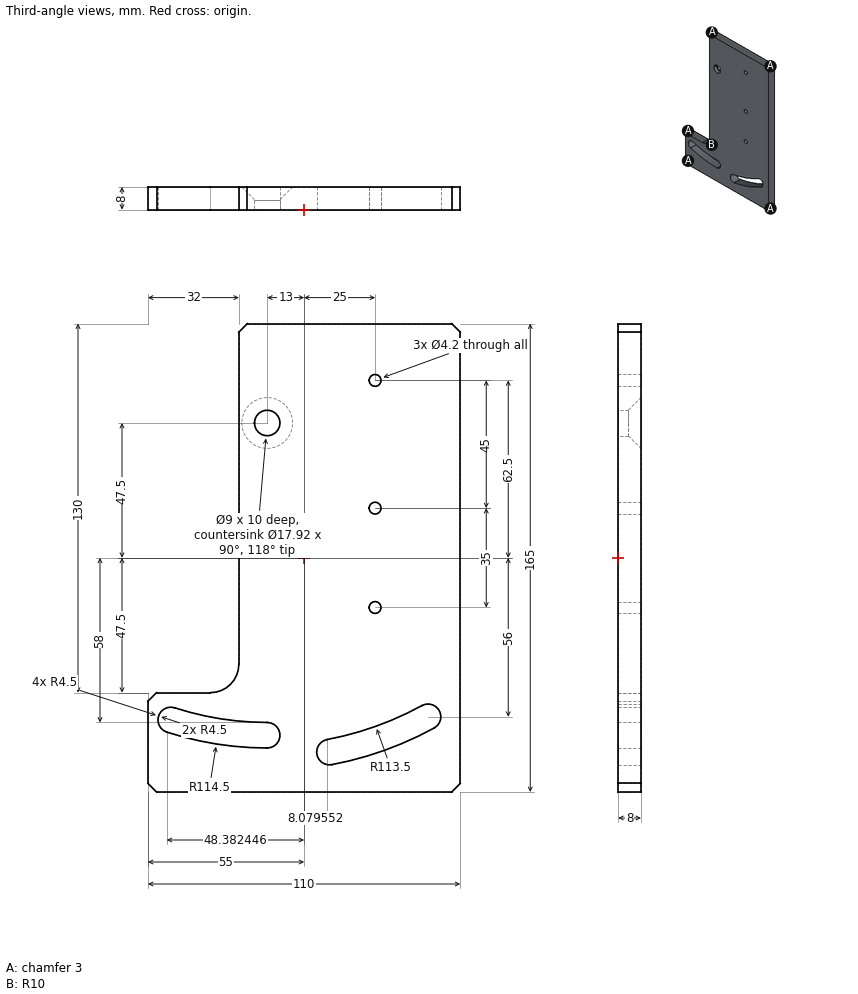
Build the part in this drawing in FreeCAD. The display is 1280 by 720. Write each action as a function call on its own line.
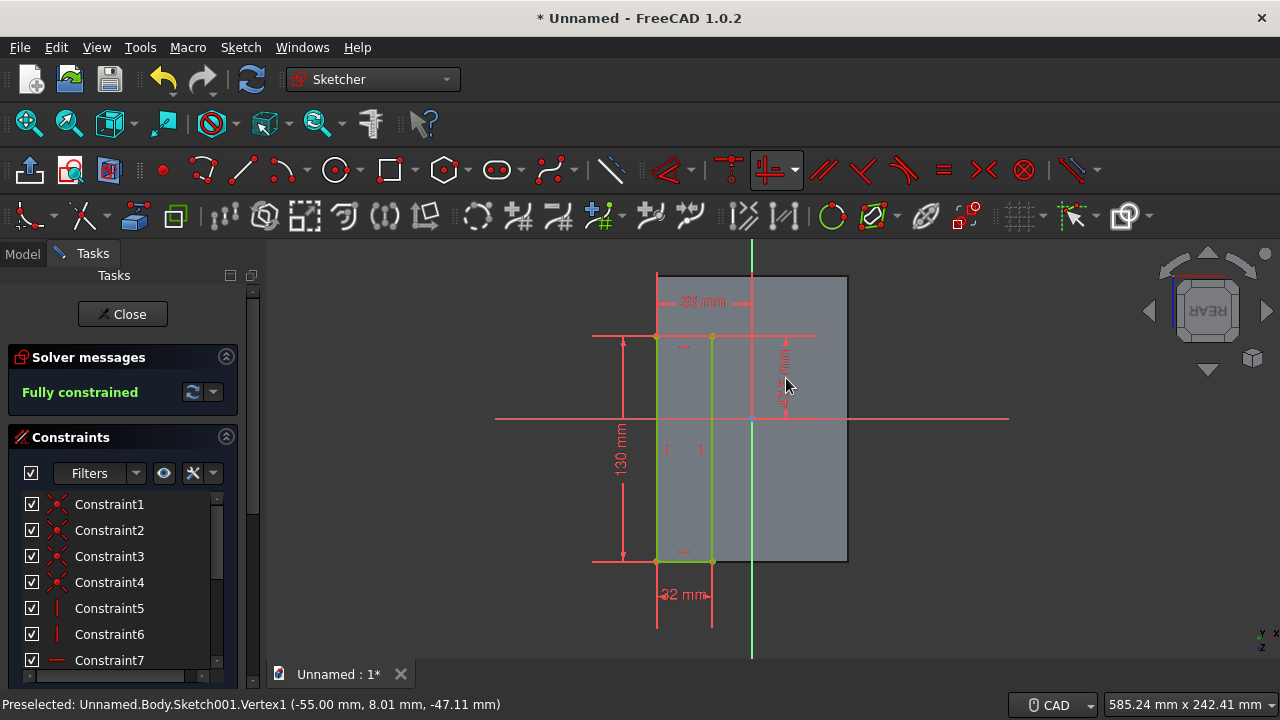
click(123, 314)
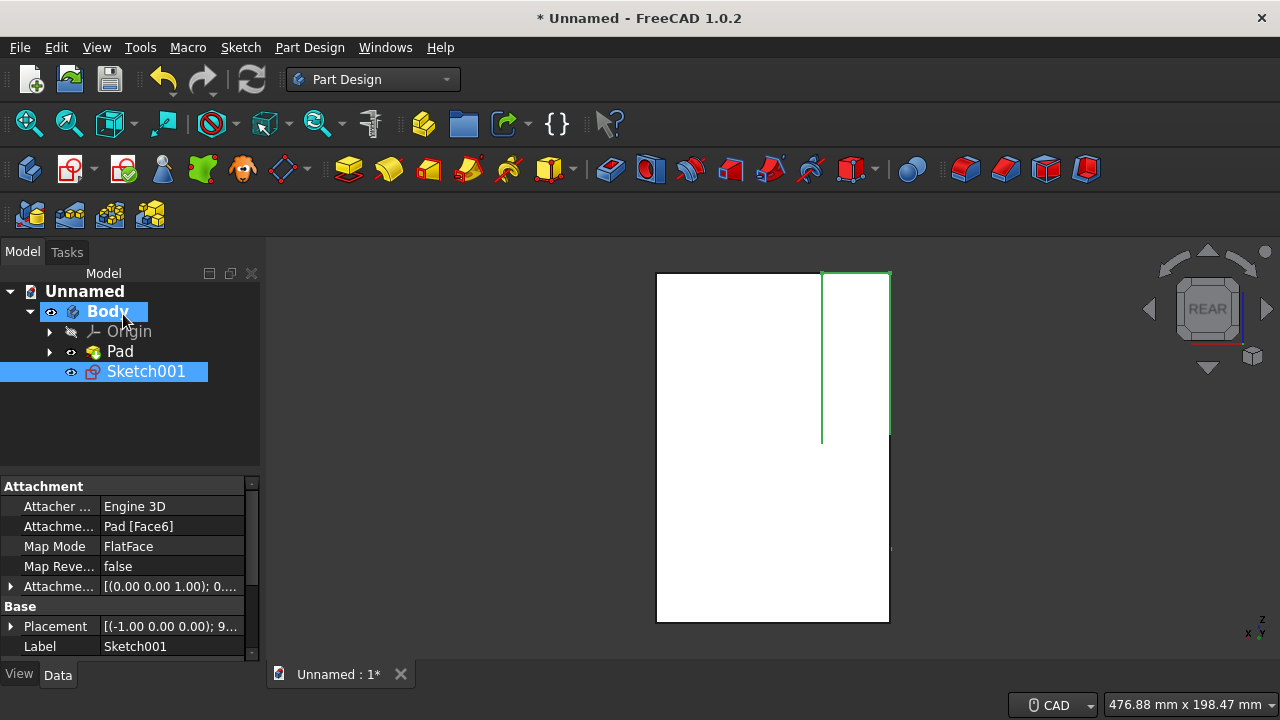
click(612, 170)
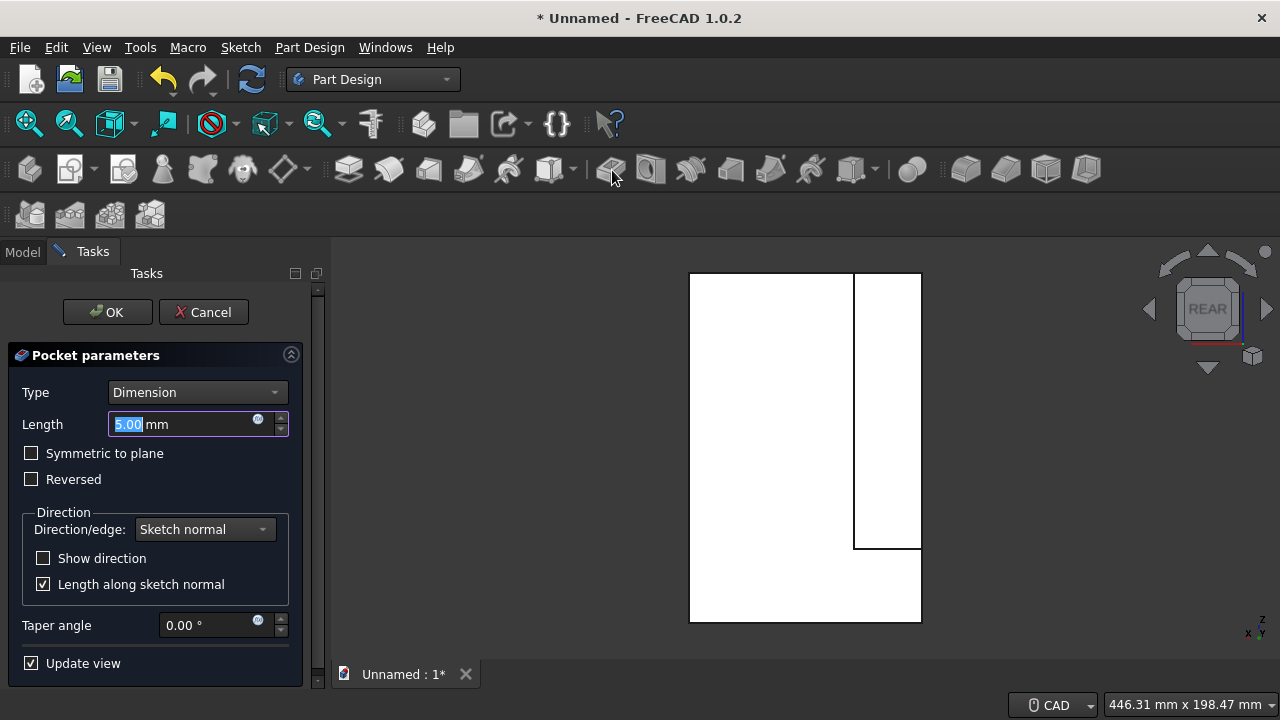
text(8)
key(Tab)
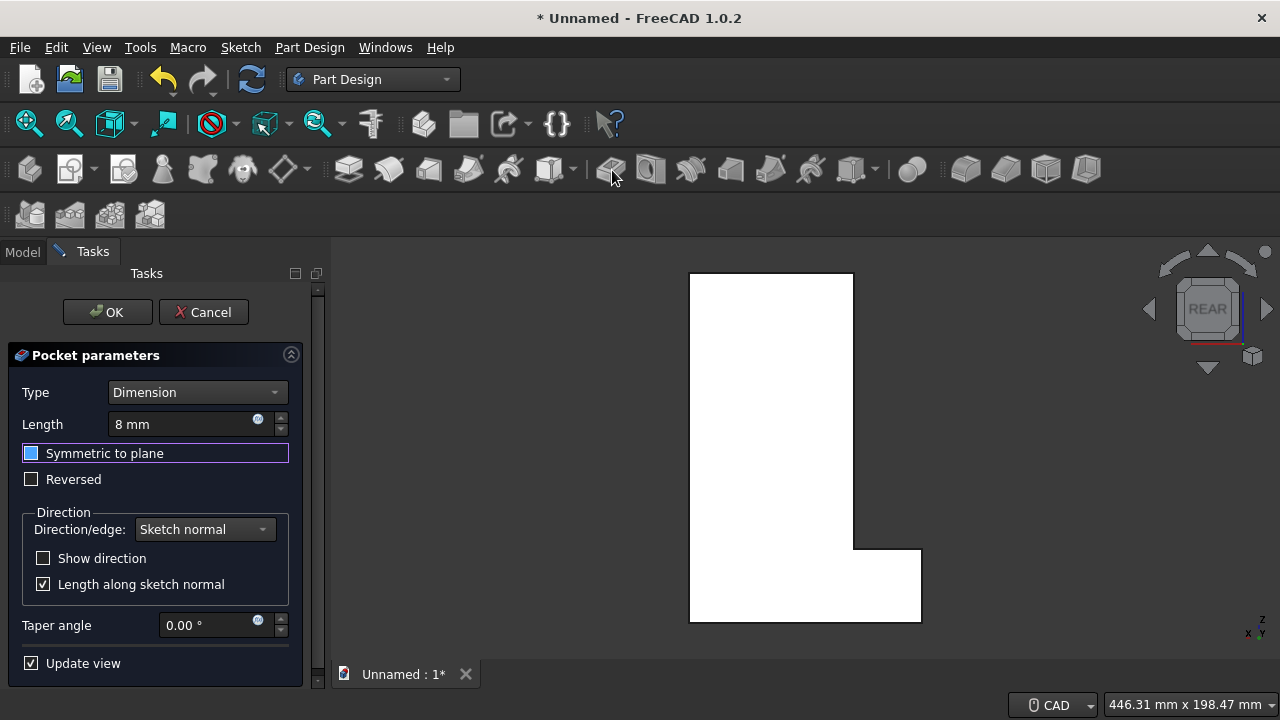
click(108, 312)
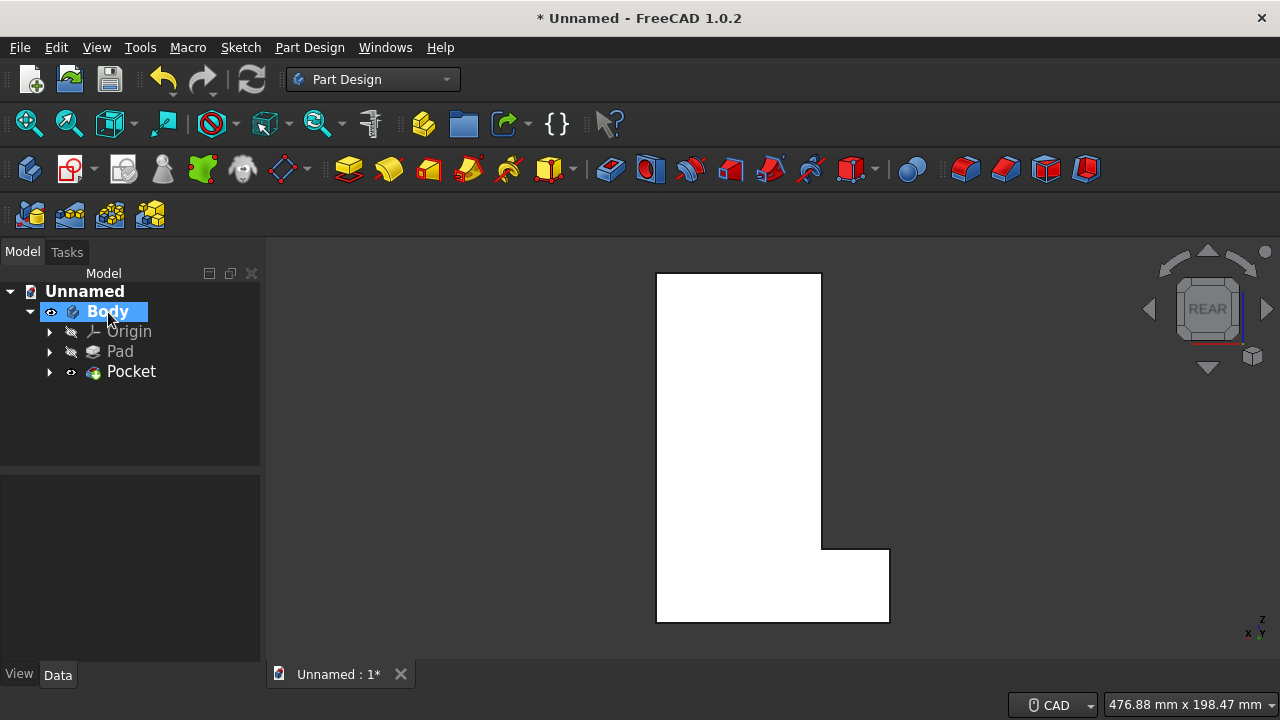
click(740, 397)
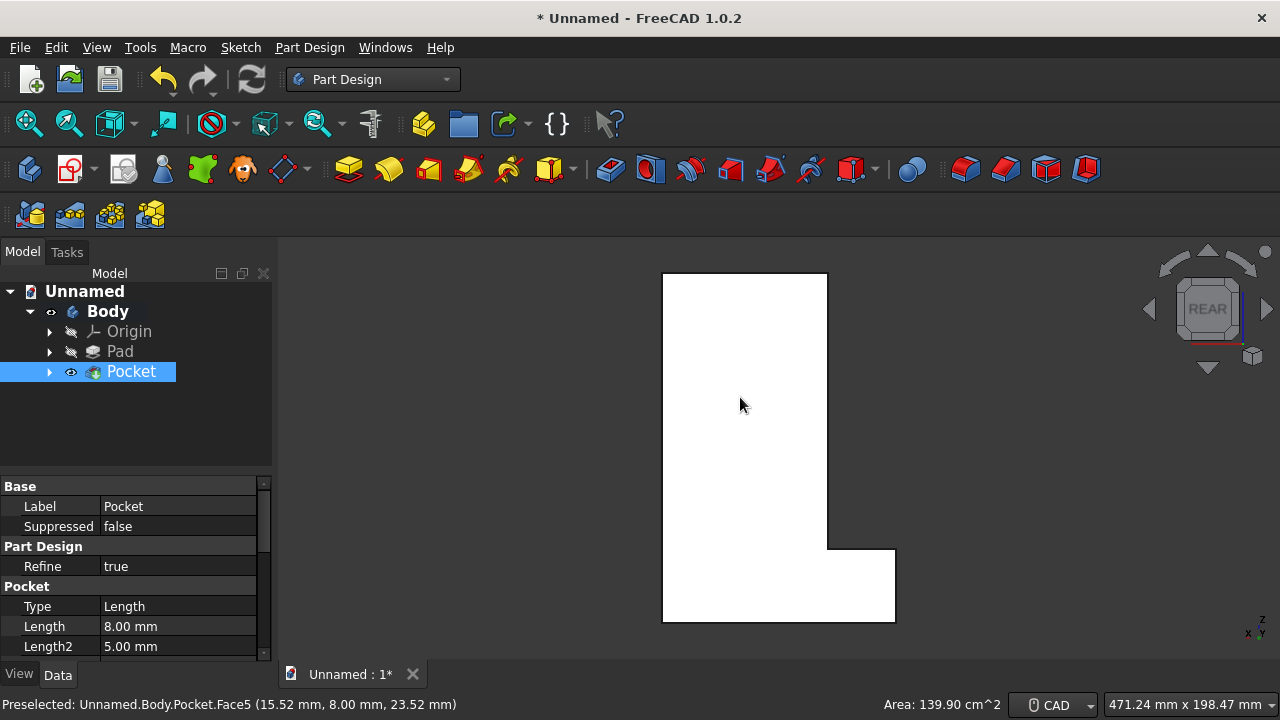
click(70, 170)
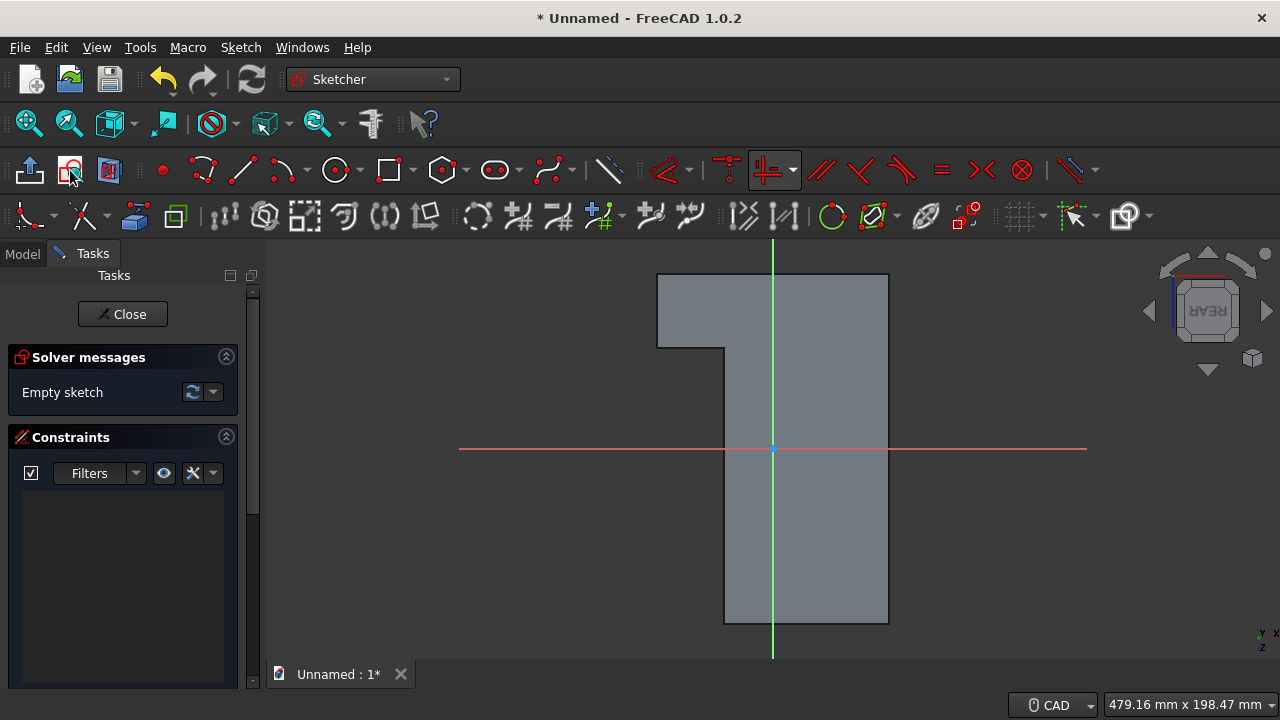
scroll(749, 558, up, 13)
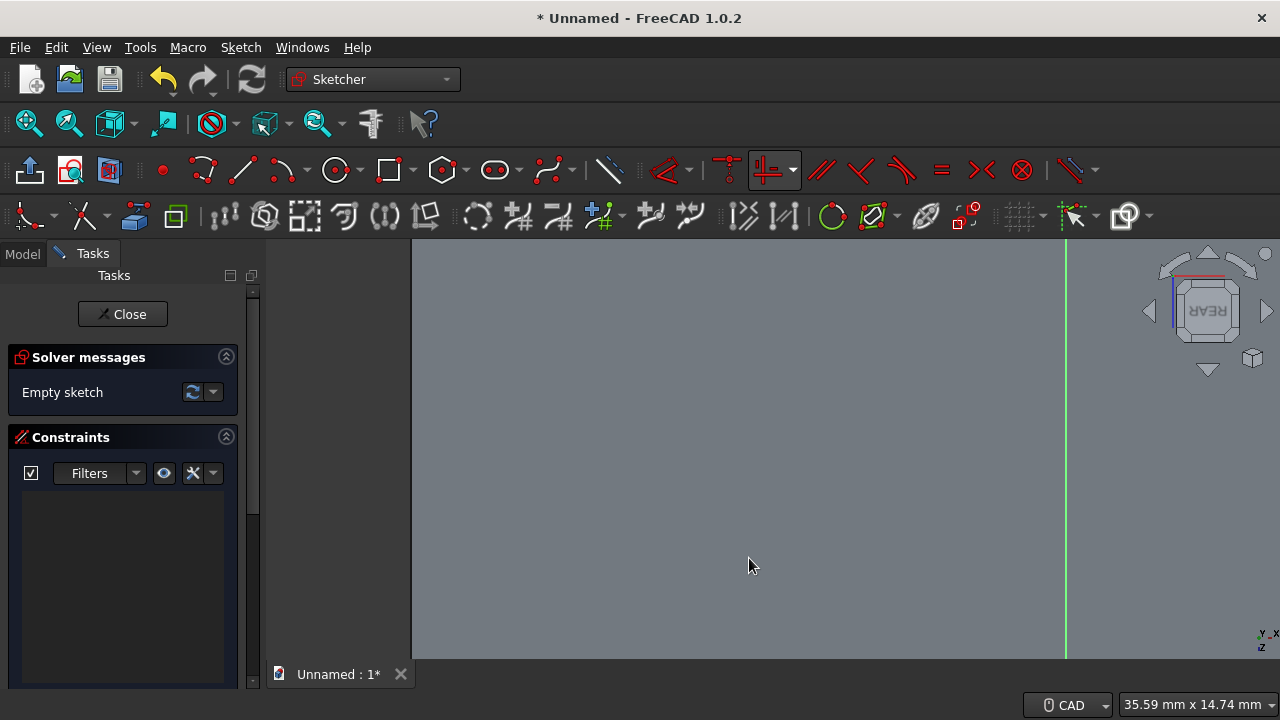
click(336, 170)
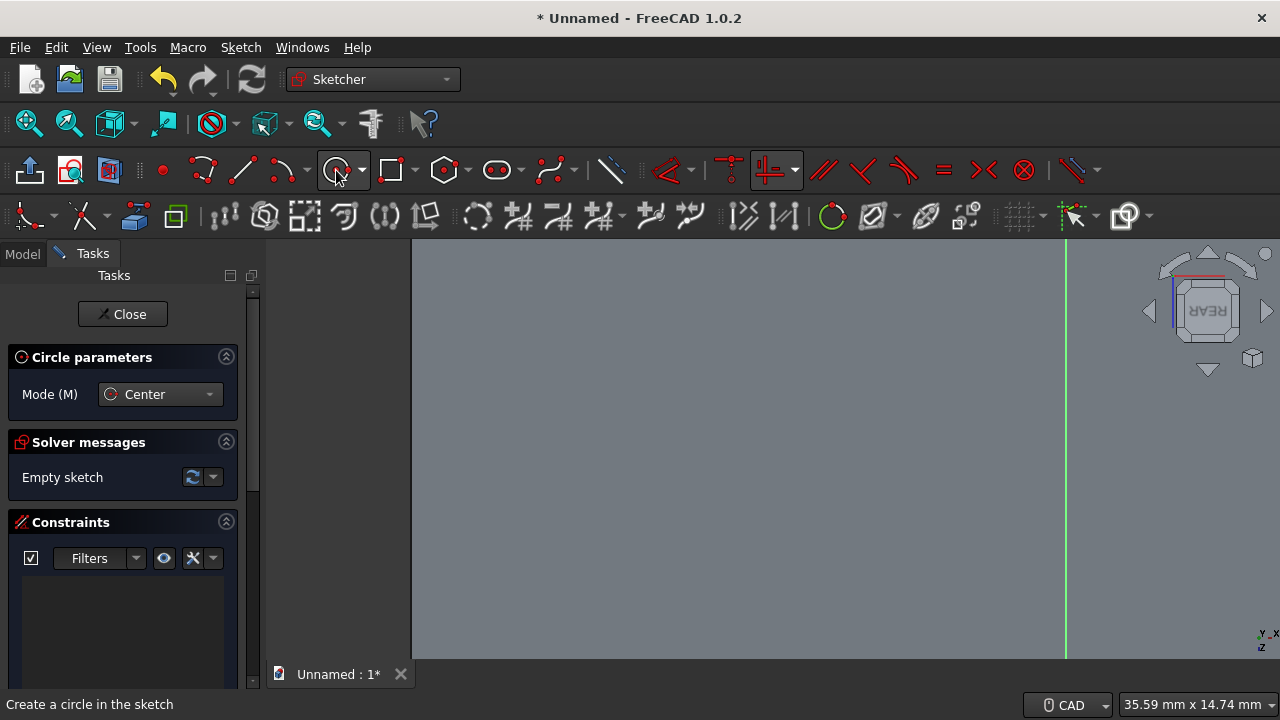
click(696, 434)
click(786, 344)
key(Escape)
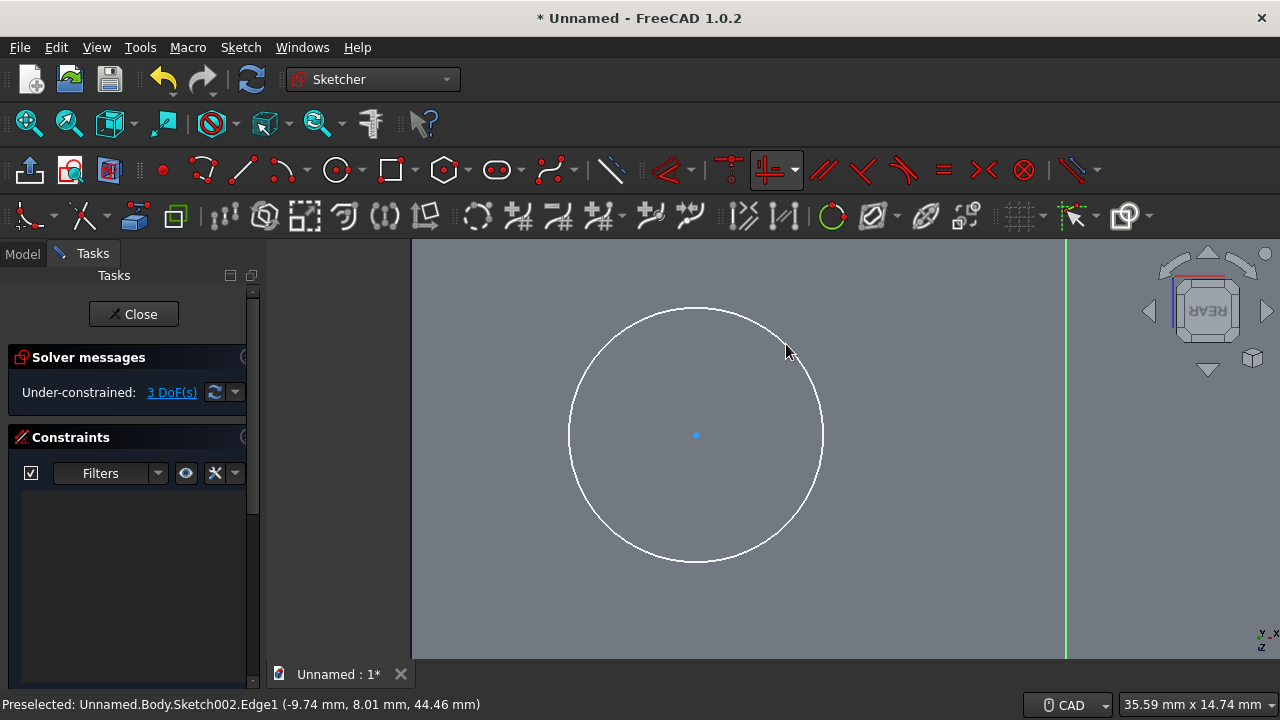
click(666, 170)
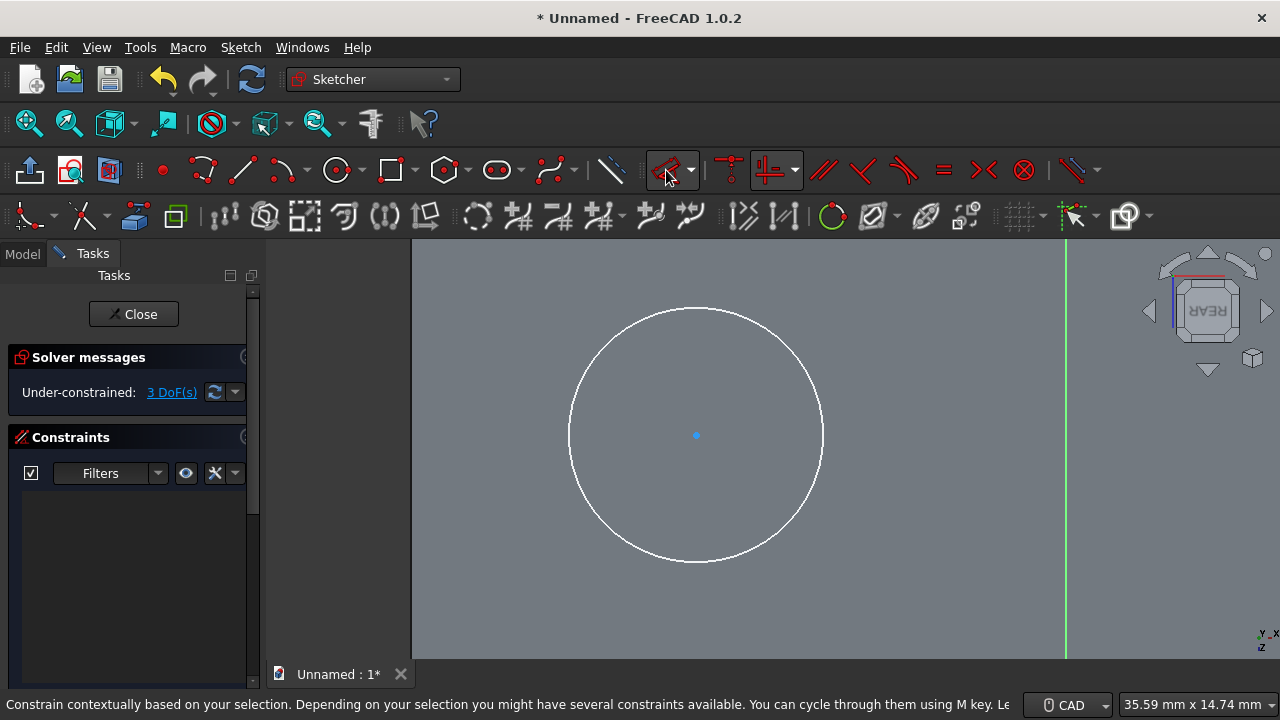
click(786, 345)
click(809, 322)